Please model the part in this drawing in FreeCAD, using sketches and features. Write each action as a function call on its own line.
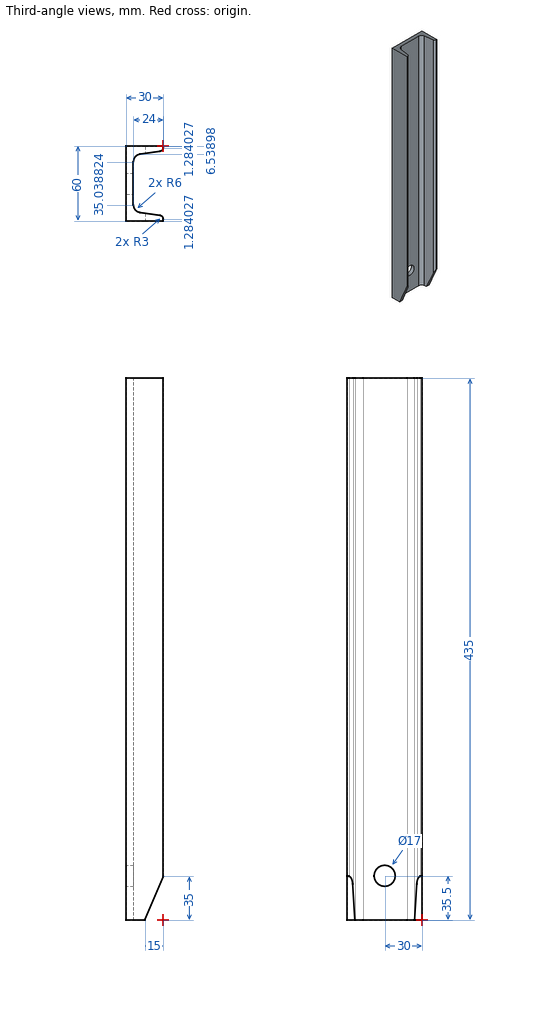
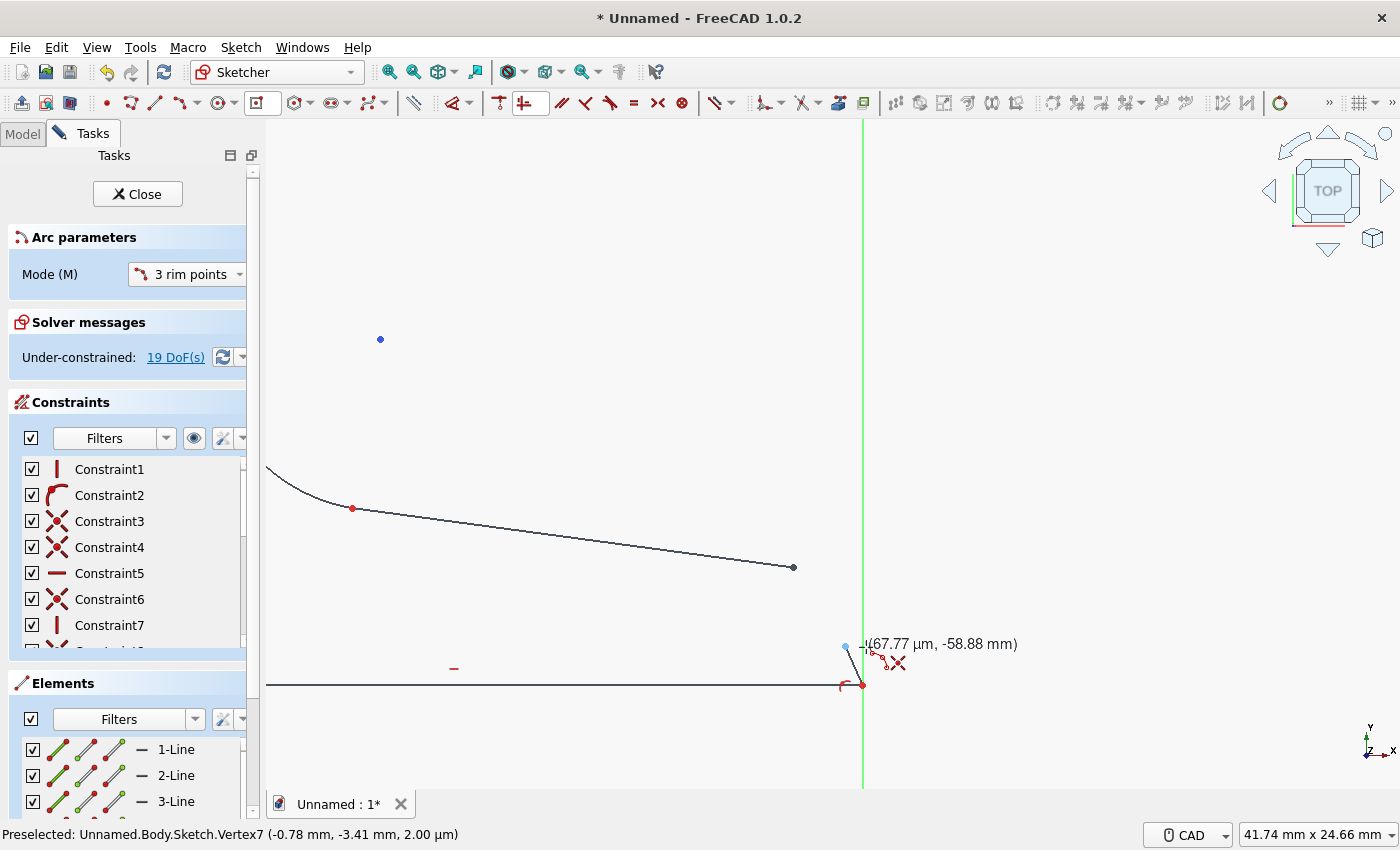
click(845, 646)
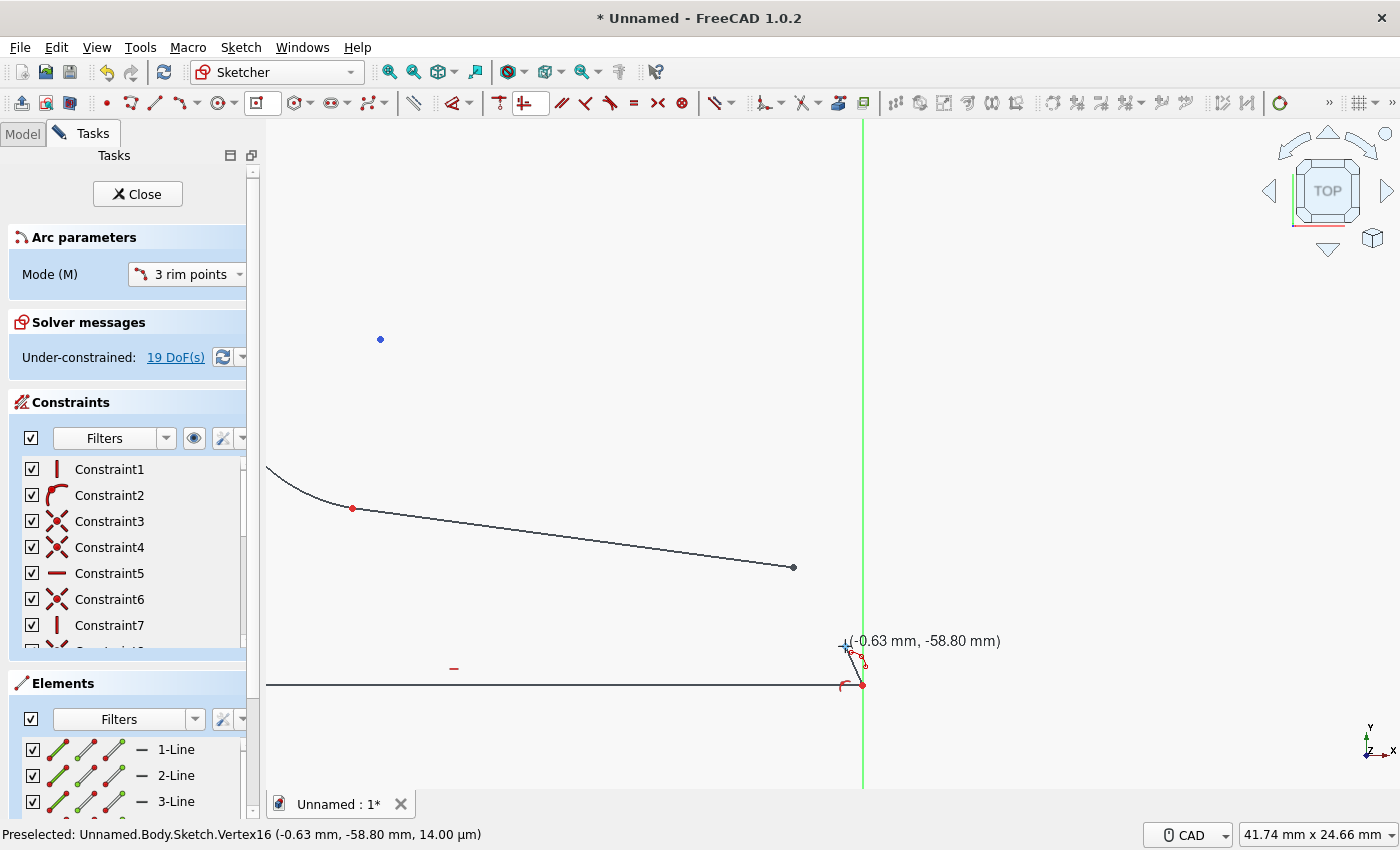
scroll(866, 647, down, 7)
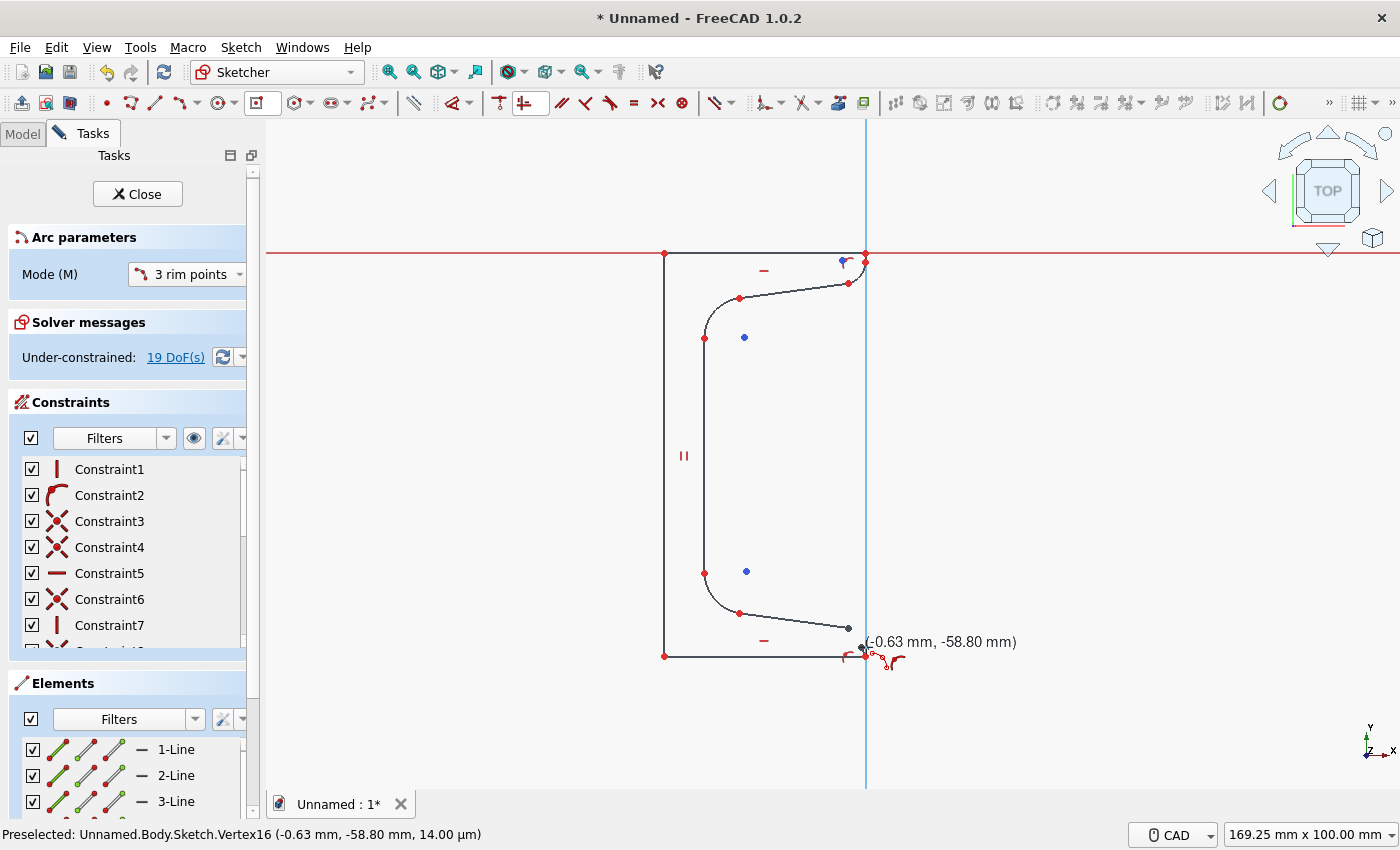
click(849, 628)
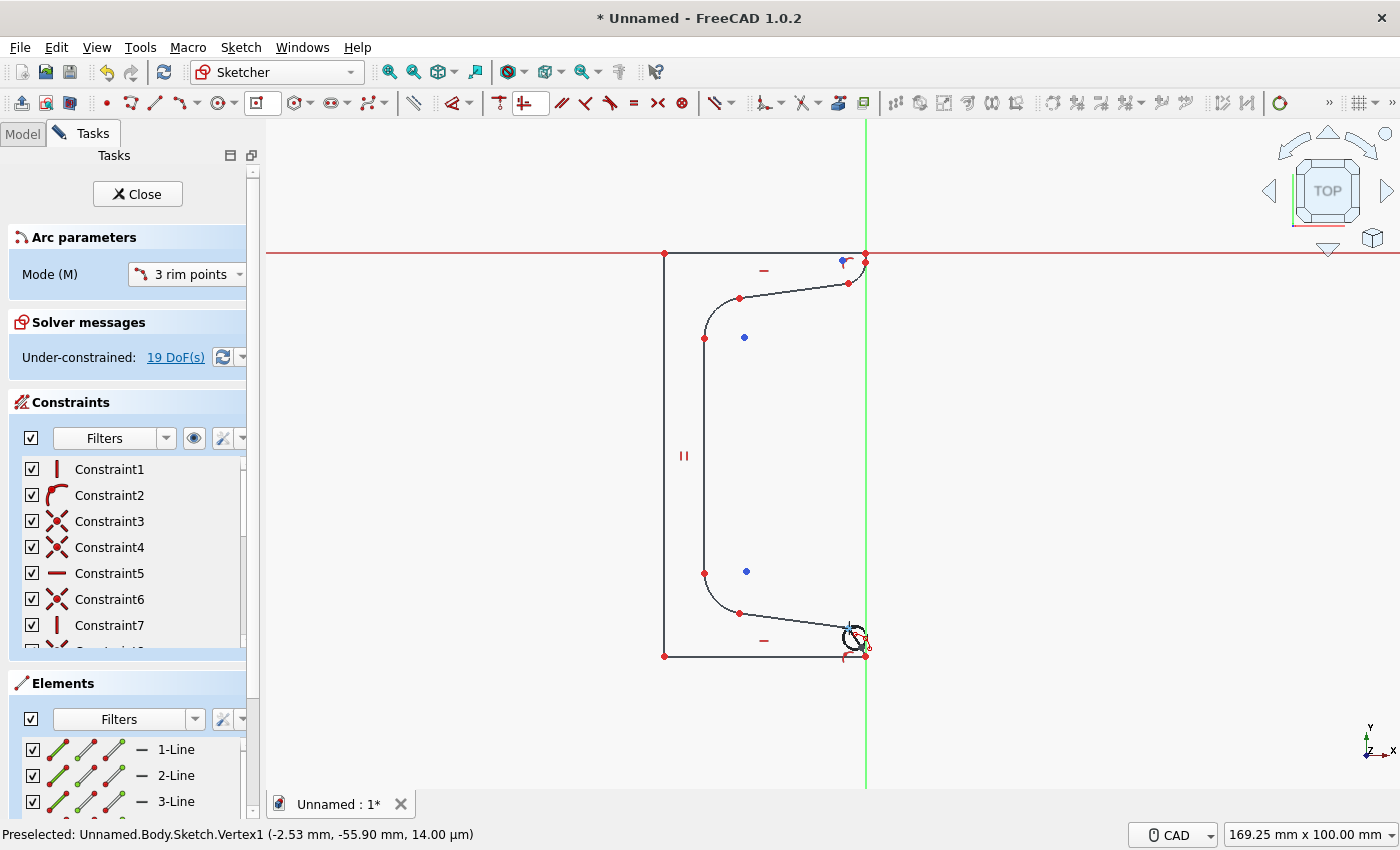
scroll(861, 634, up, 6)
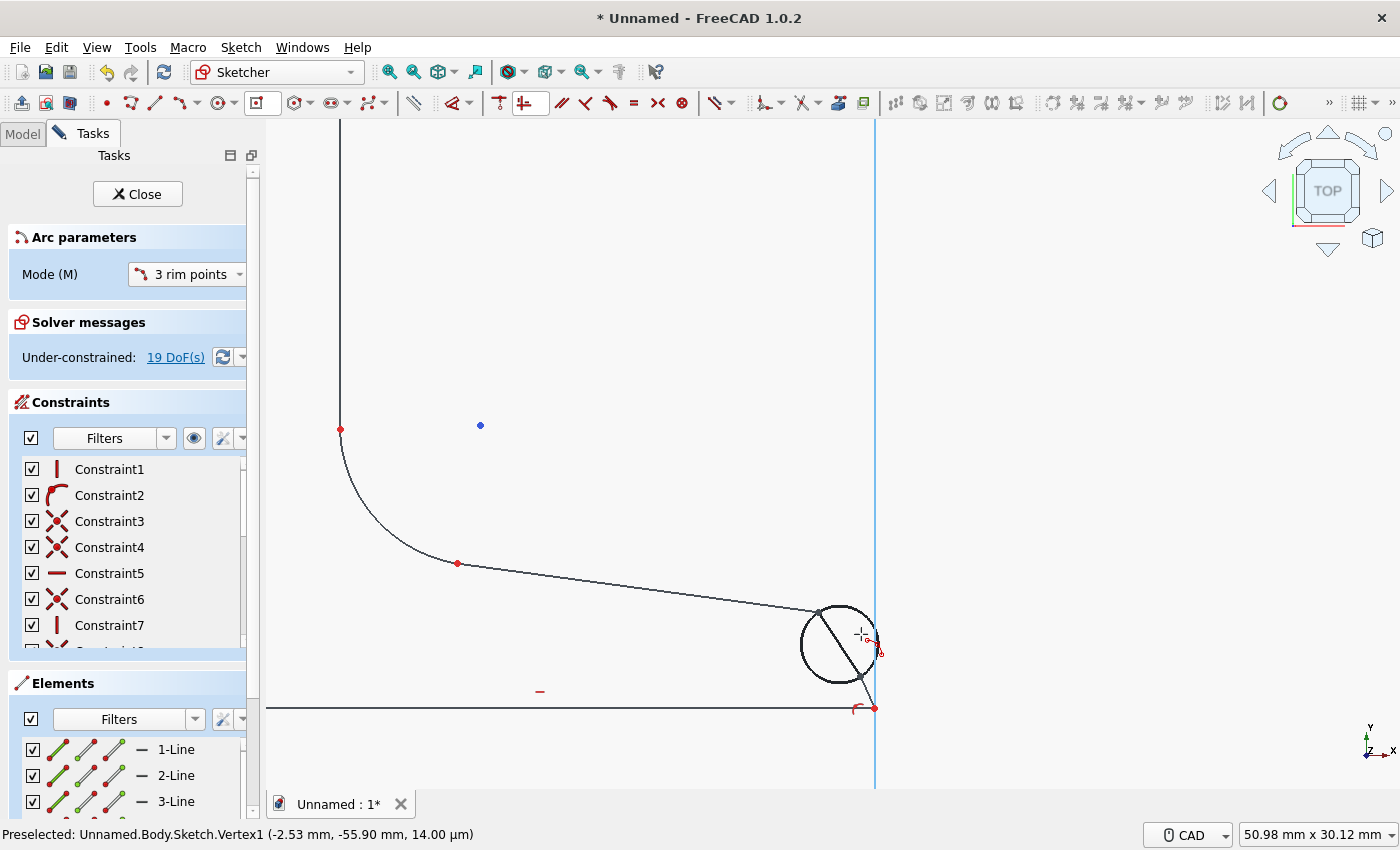
click(859, 631)
key(Escape)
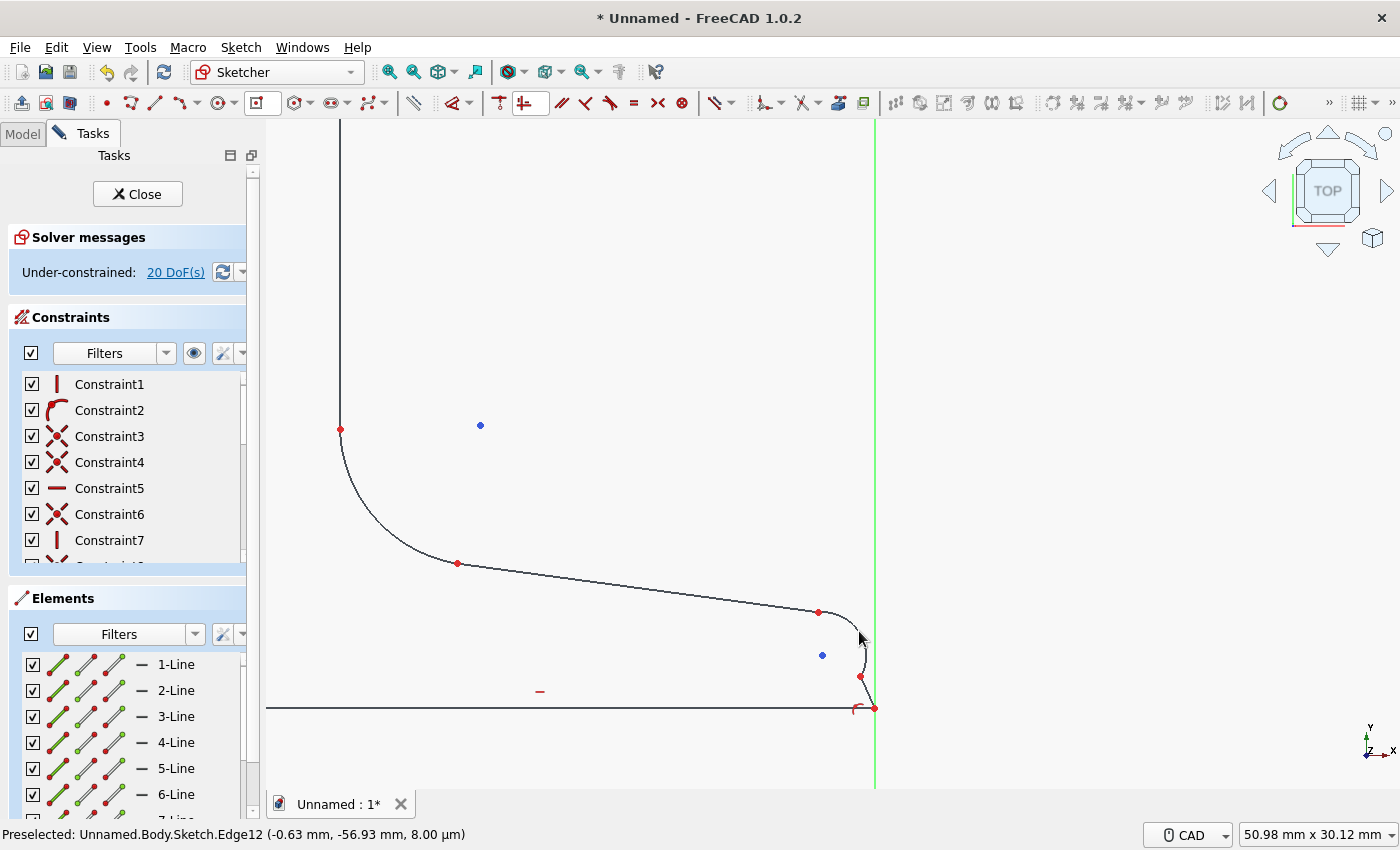
scroll(861, 634, down, 6)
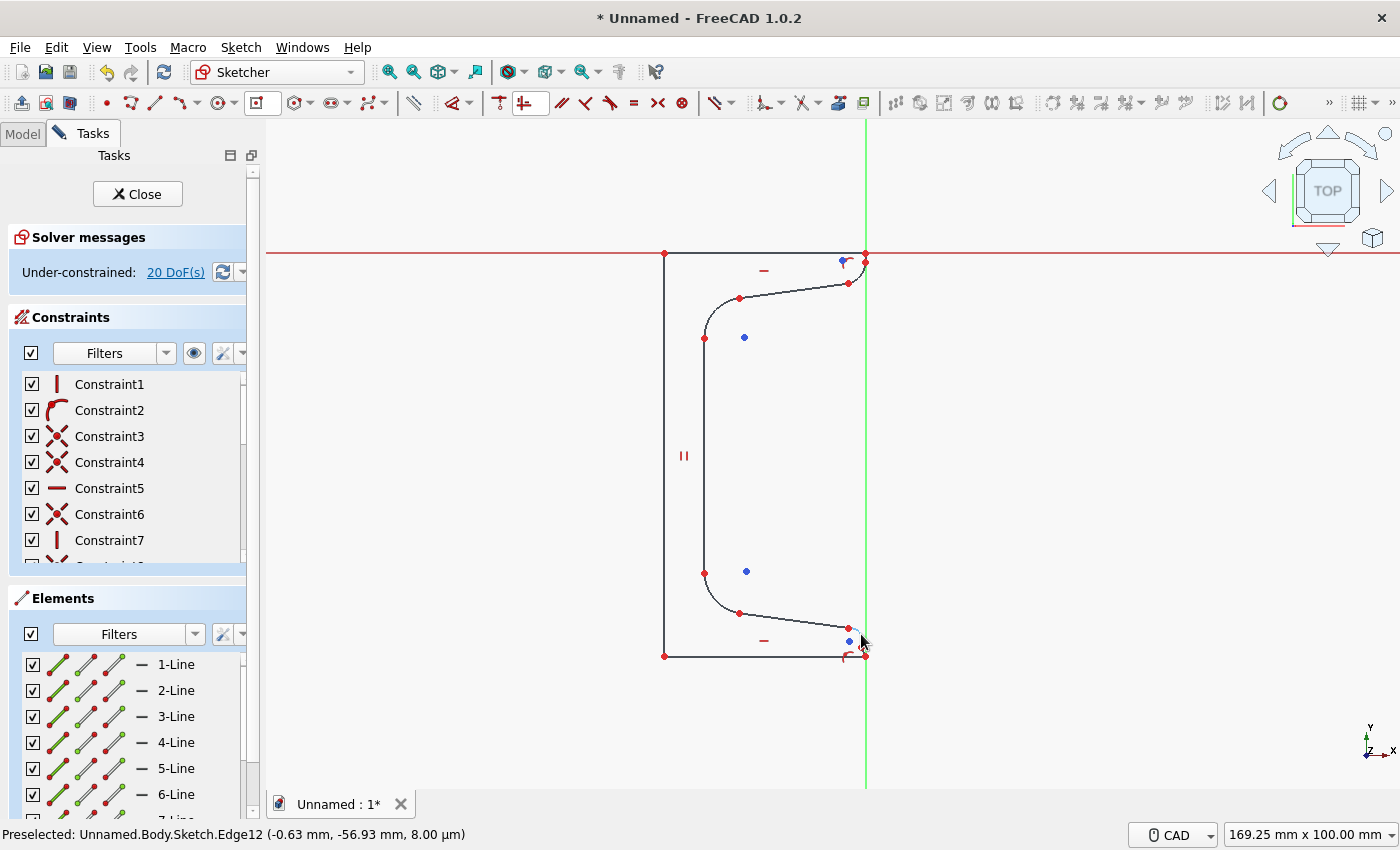
click(816, 624)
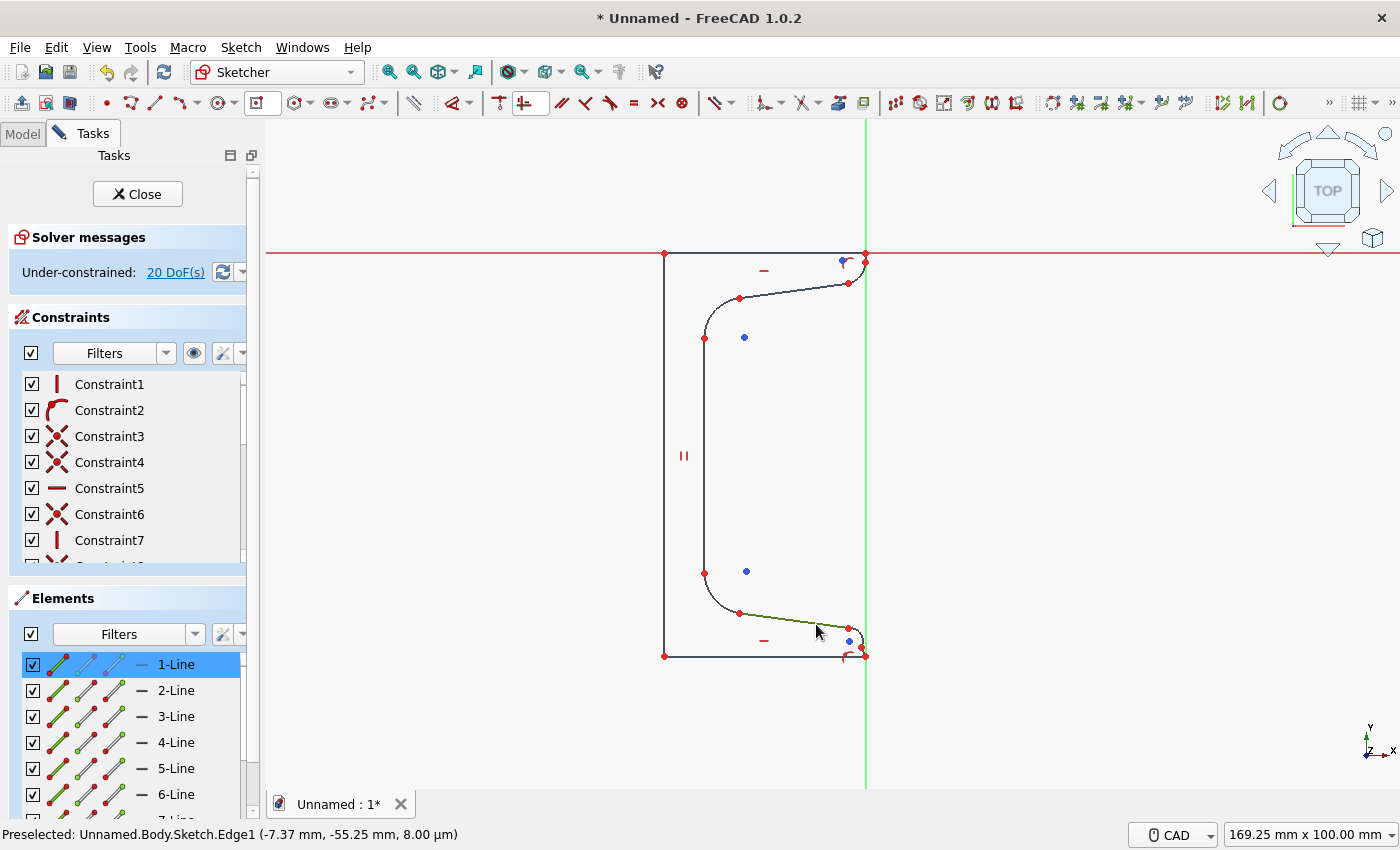
click(709, 590)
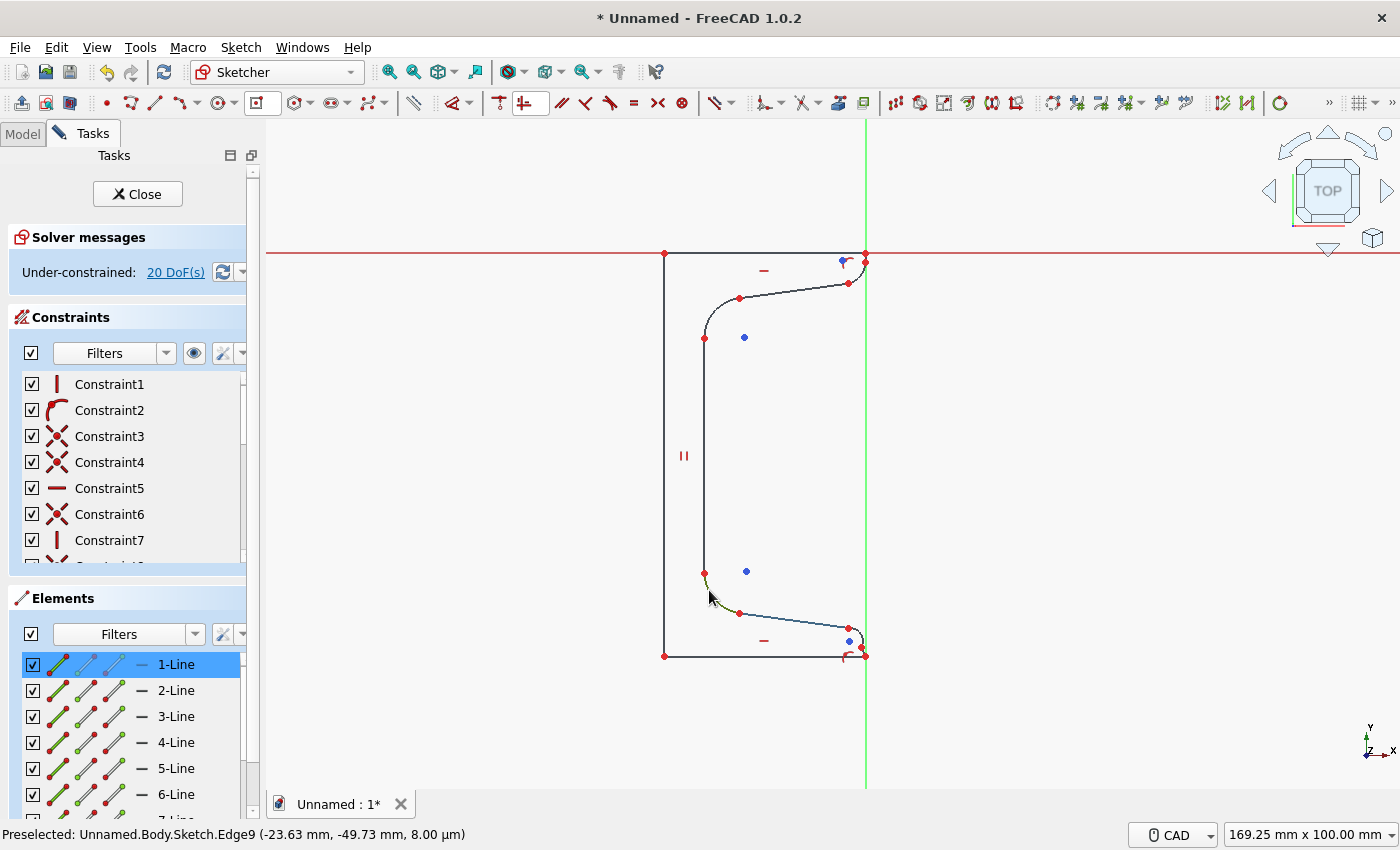
click(610, 104)